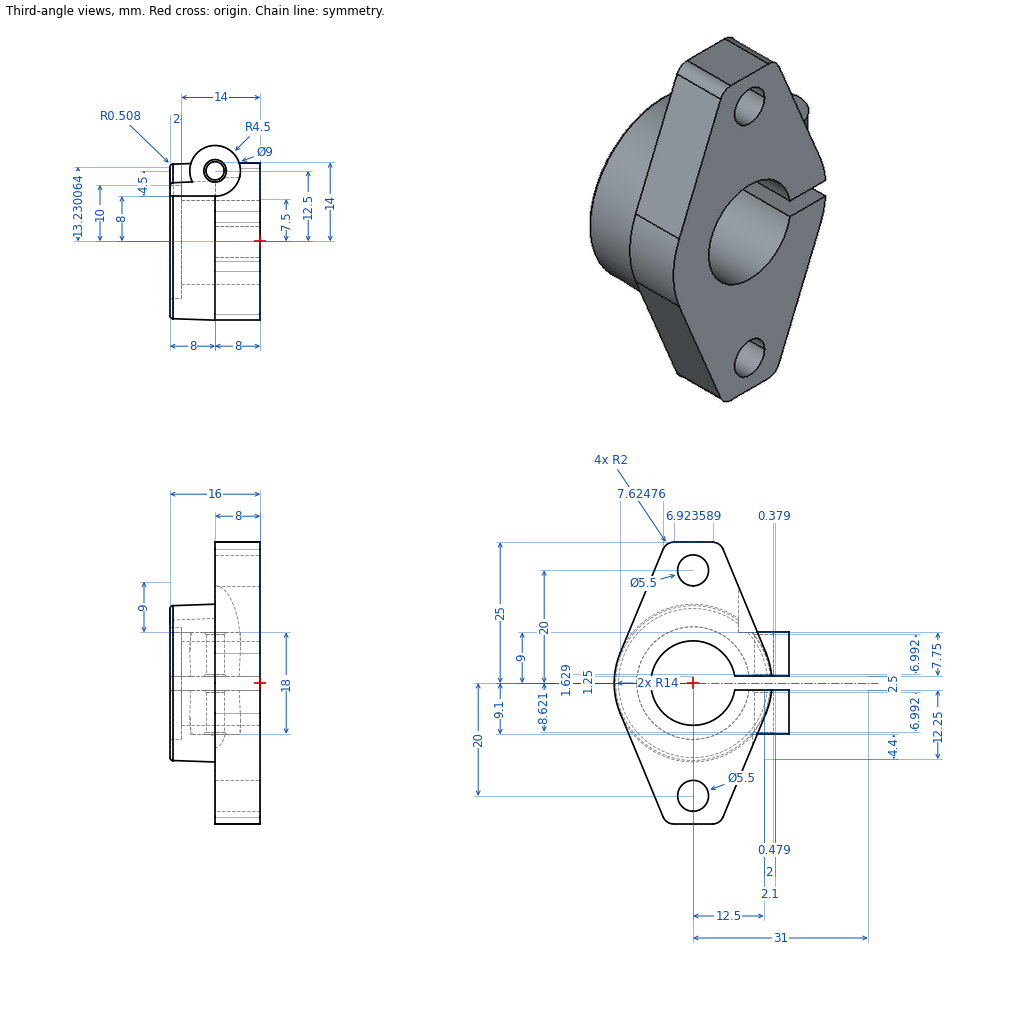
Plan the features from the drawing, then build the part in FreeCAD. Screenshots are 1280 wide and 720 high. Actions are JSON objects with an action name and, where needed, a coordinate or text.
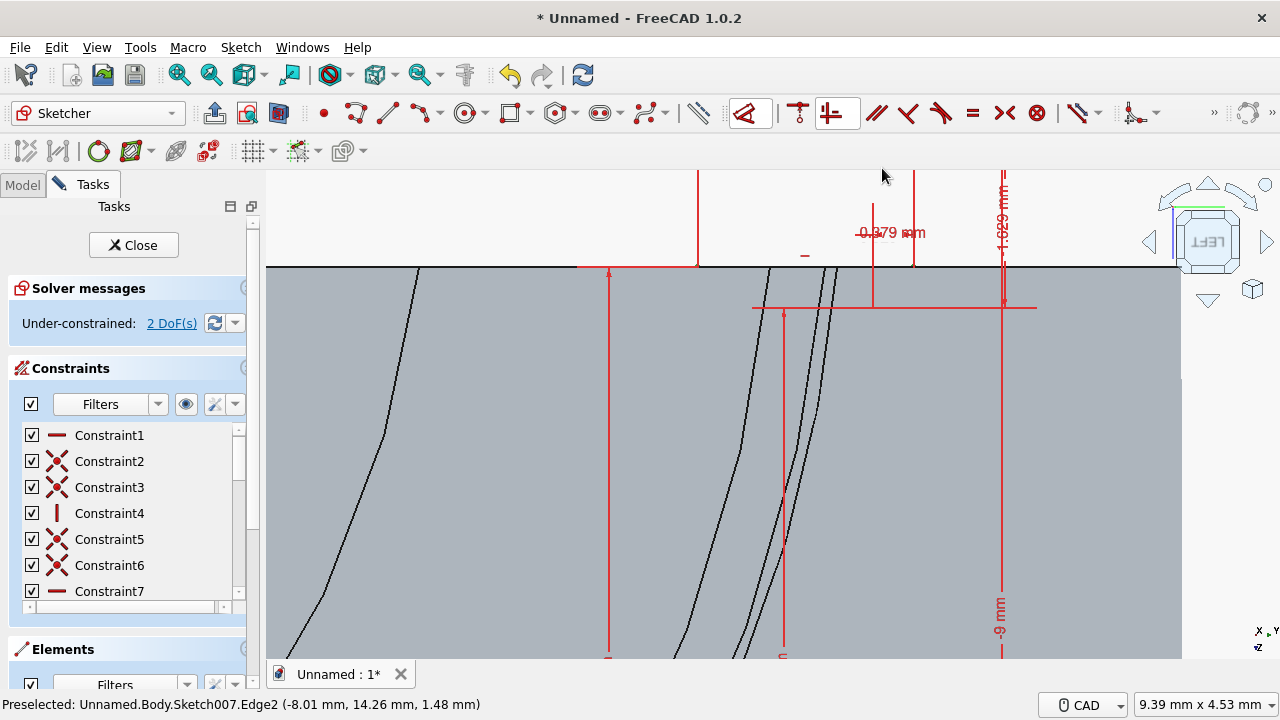
{"action": "left_click", "coordinate": [134, 245]}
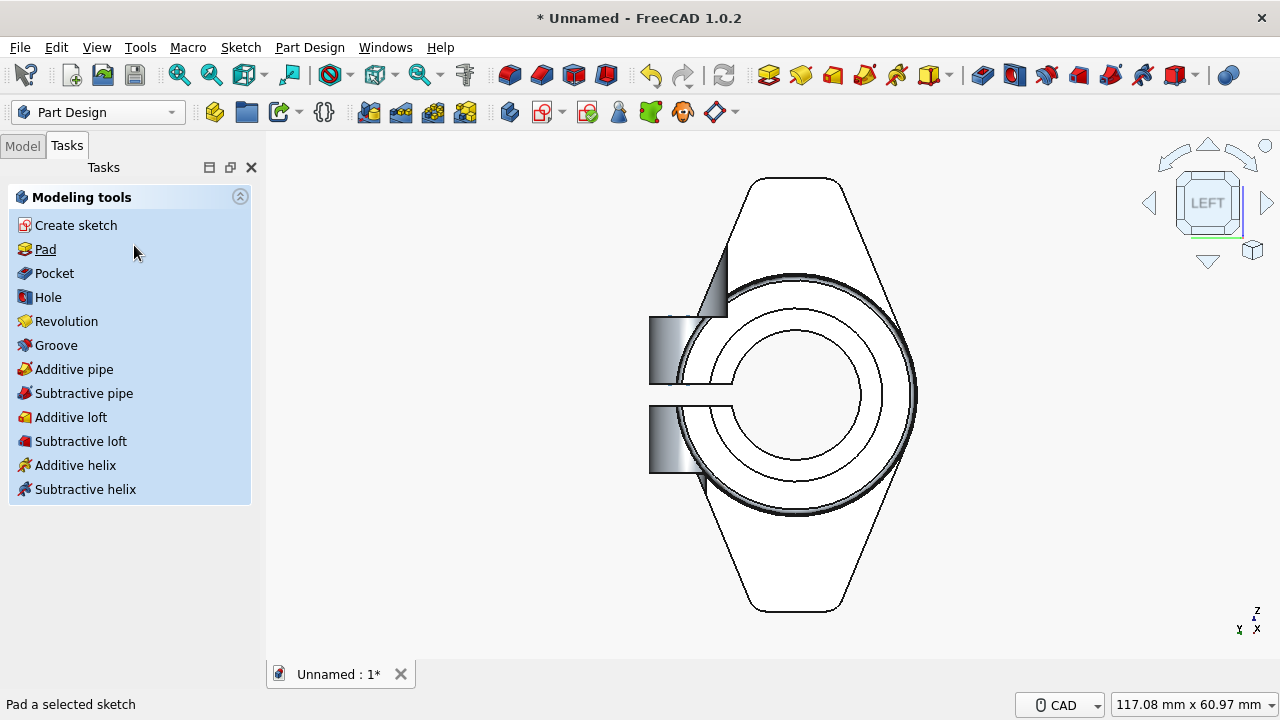
{"action": "left_click", "coordinate": [1048, 76]}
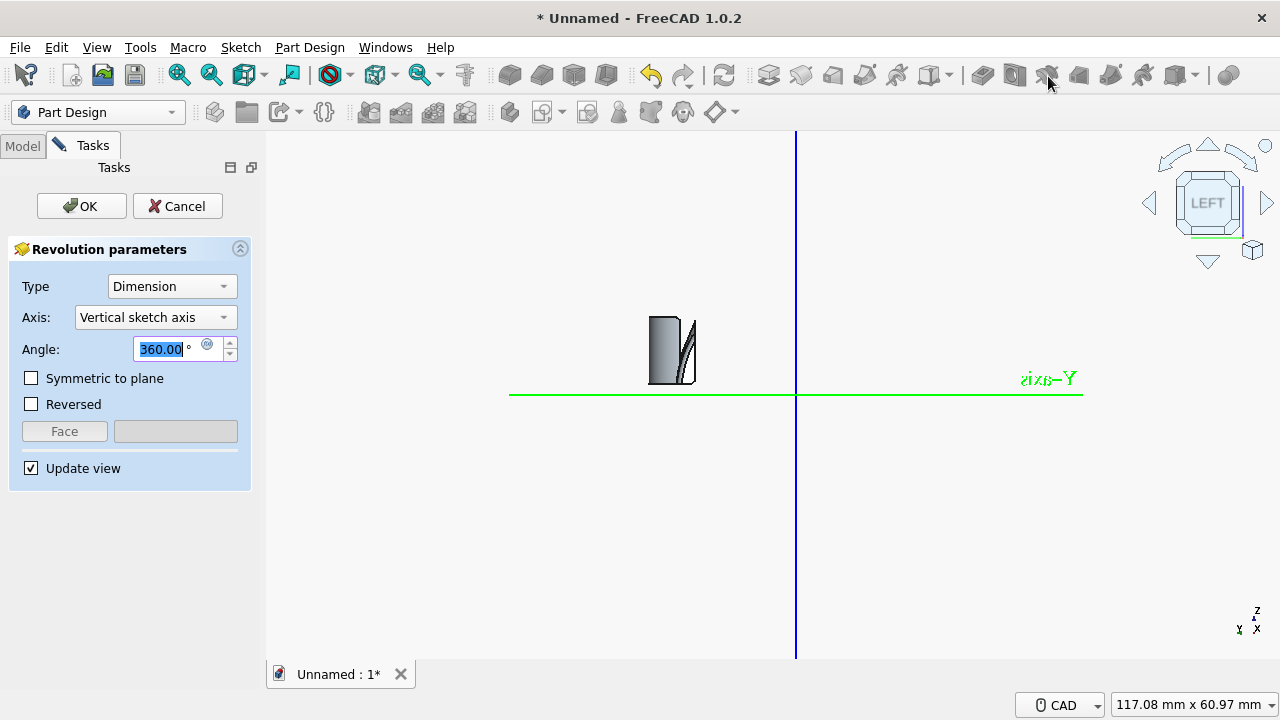
{"action": "left_click", "coordinate": [156, 318]}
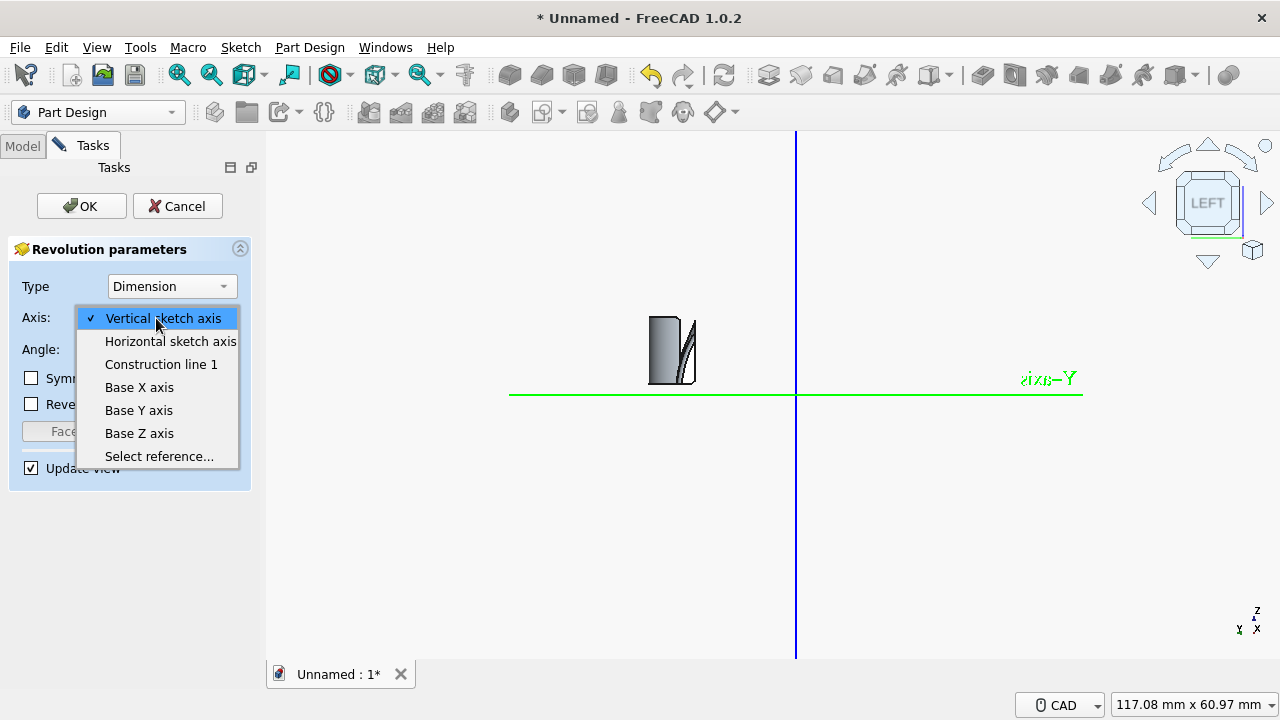
{"action": "left_click", "coordinate": [156, 364]}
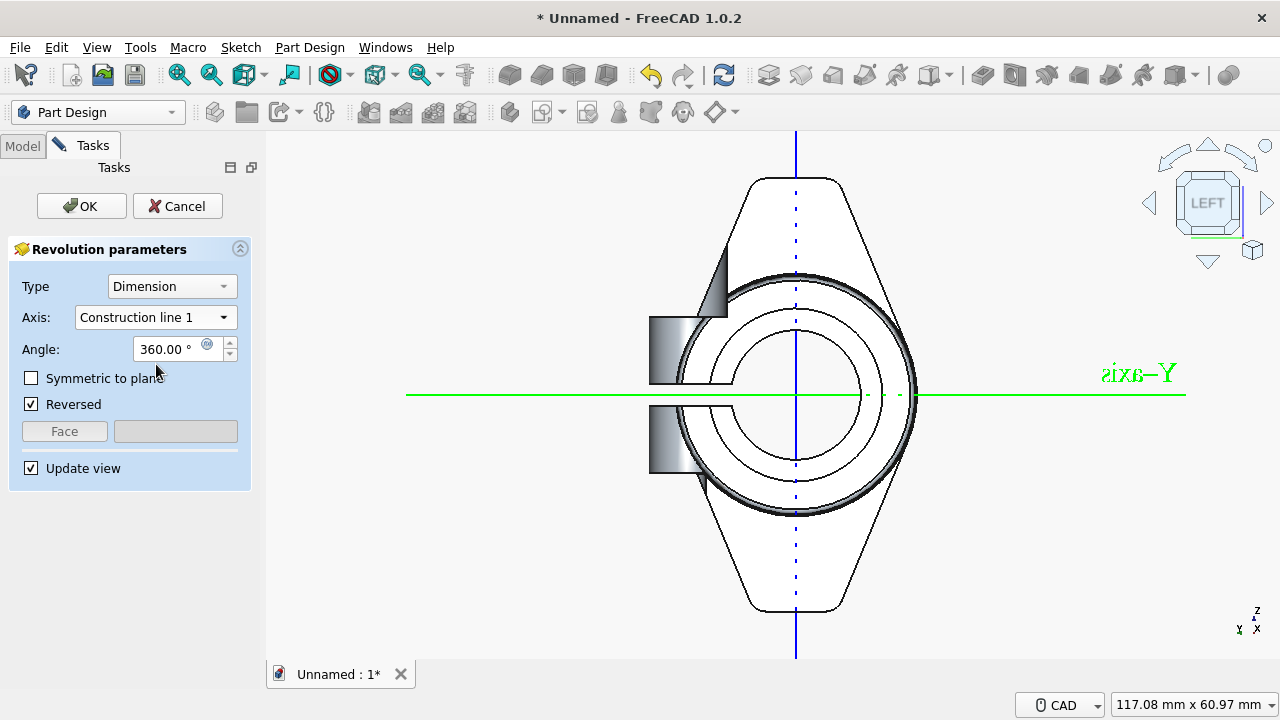
{"action": "left_click", "coordinate": [82, 206]}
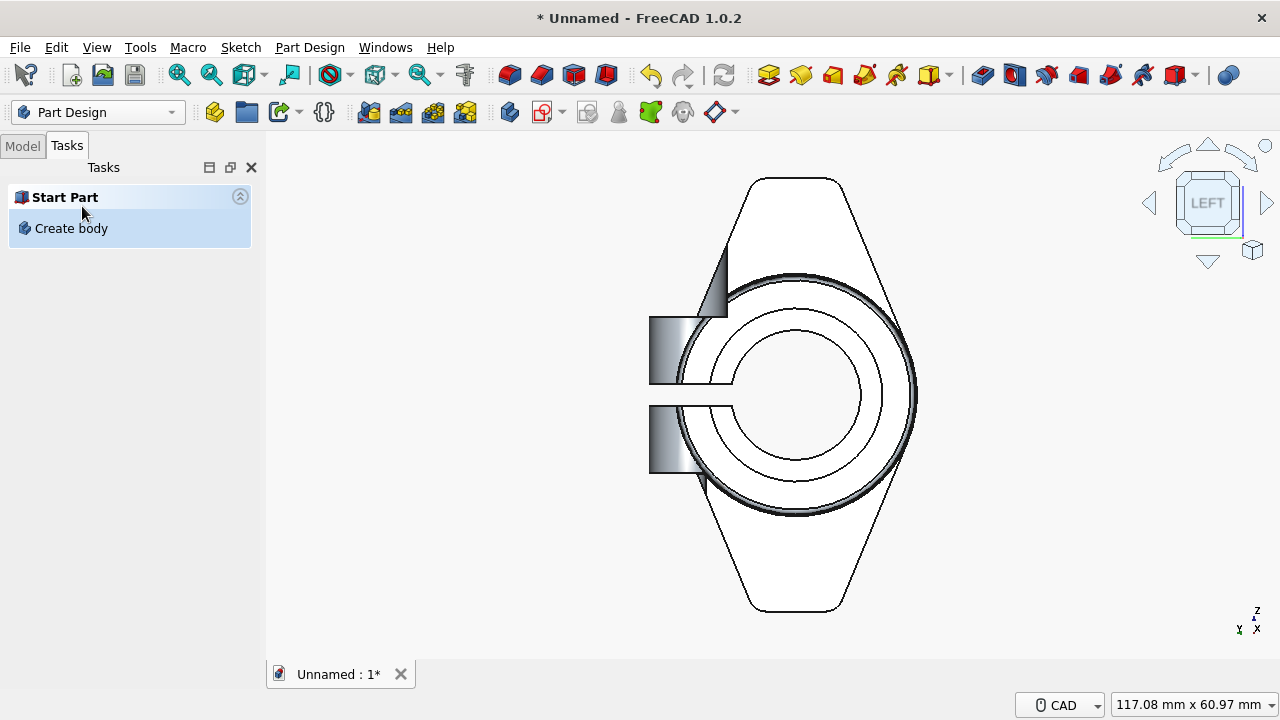
{"action": "left_click", "coordinate": [542, 112]}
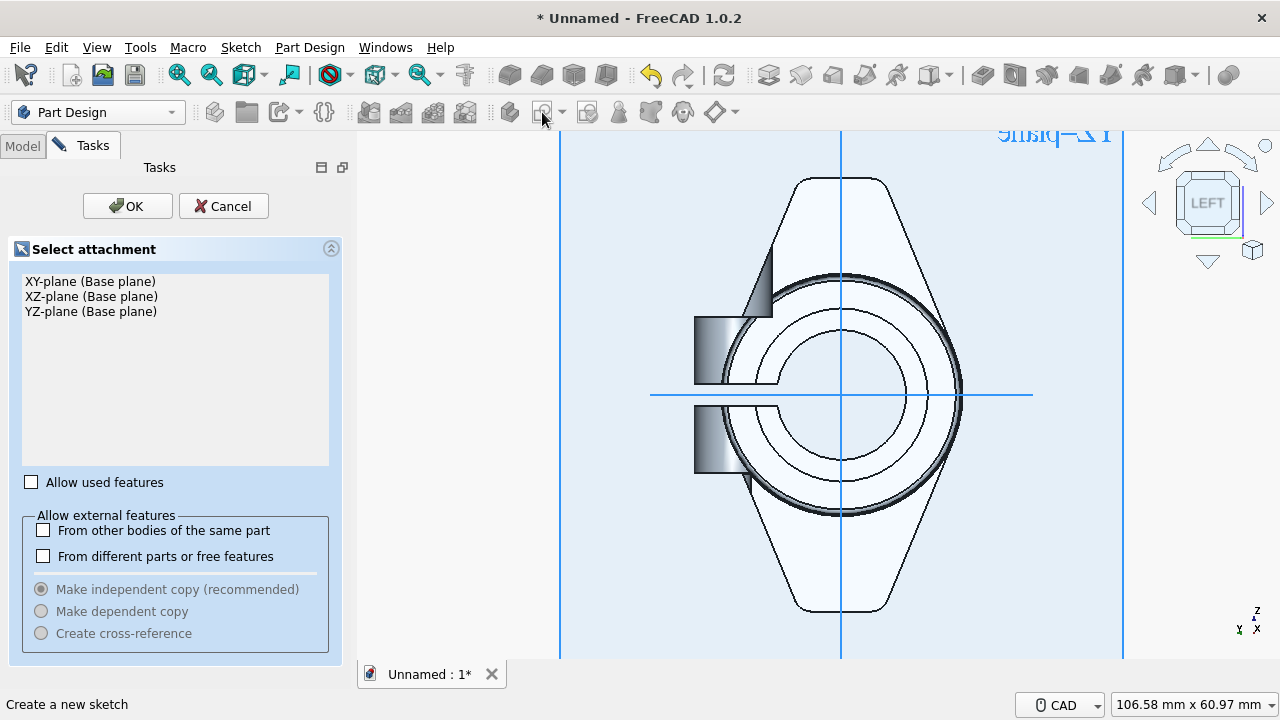
{"action": "left_click", "coordinate": [82, 312]}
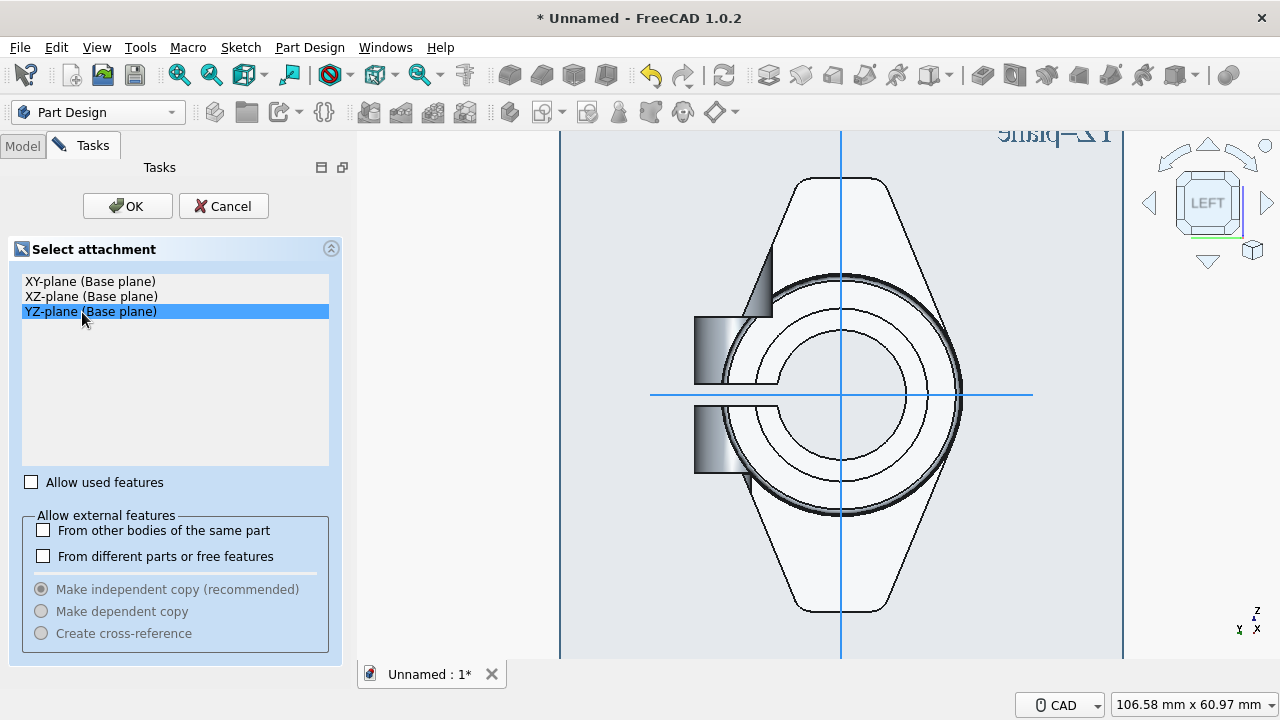
{"action": "left_click", "coordinate": [128, 206]}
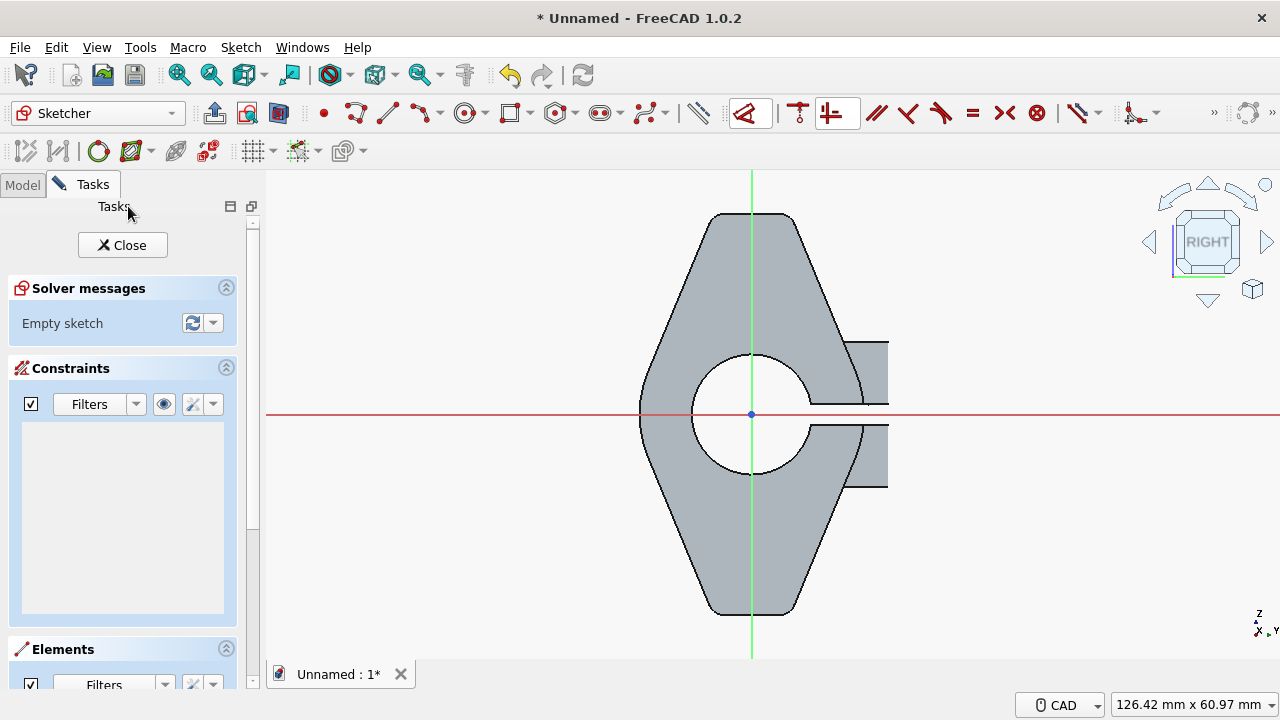
{"action": "scroll", "coordinate": [759, 600], "scroll_direction": "up", "scroll_amount": 10}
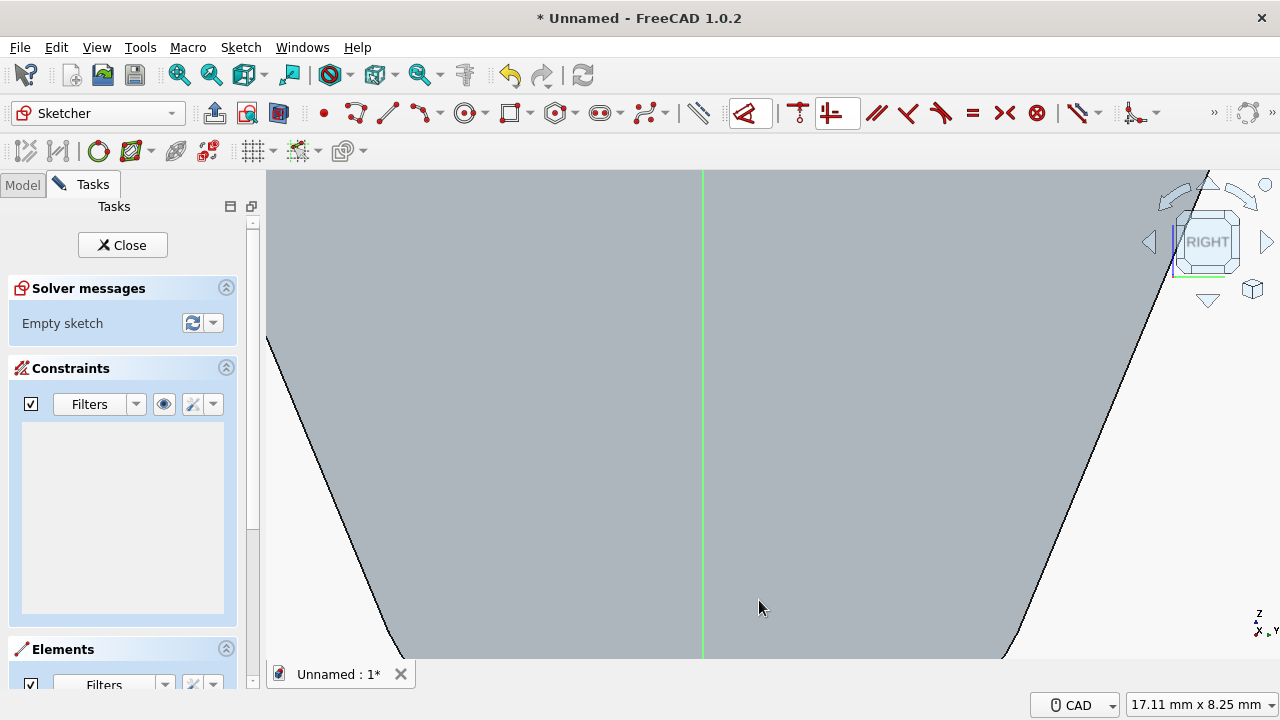
{"action": "left_click", "coordinate": [466, 114]}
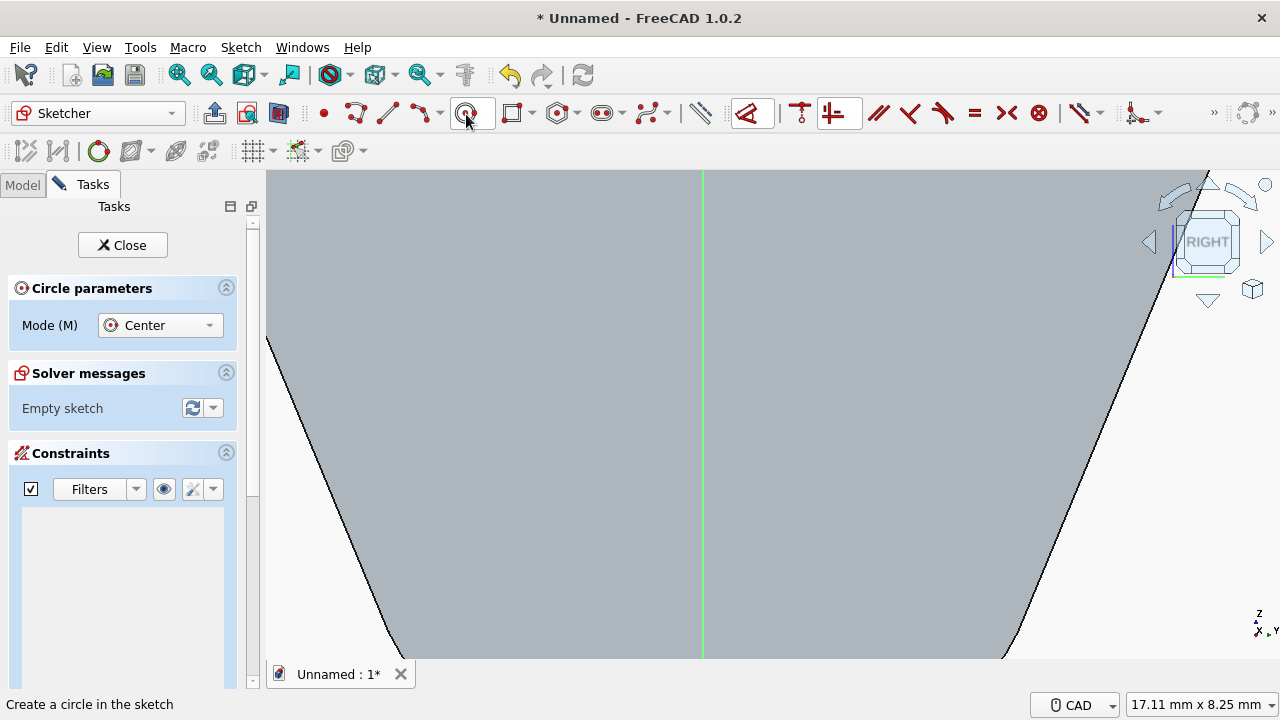
{"action": "left_click", "coordinate": [703, 409]}
{"action": "mouse_move", "coordinate": [818, 294]}